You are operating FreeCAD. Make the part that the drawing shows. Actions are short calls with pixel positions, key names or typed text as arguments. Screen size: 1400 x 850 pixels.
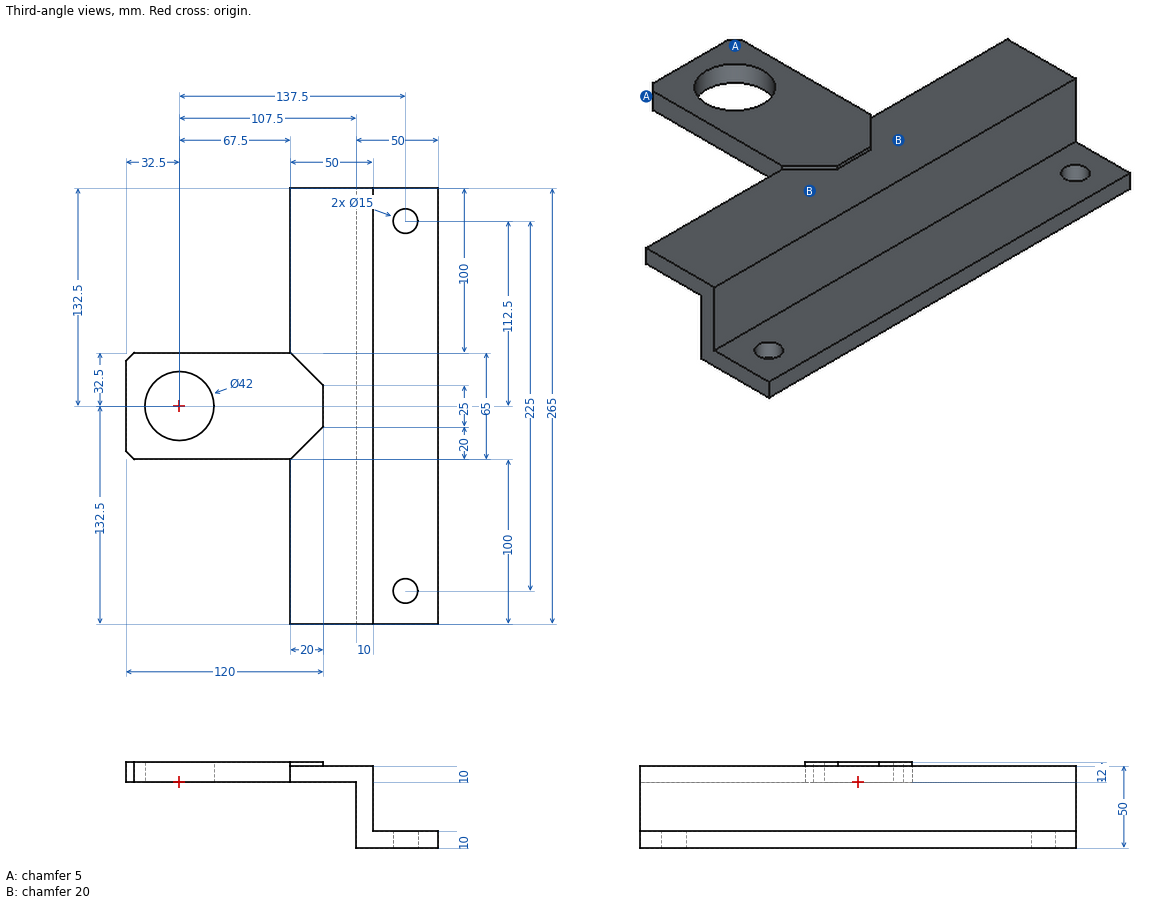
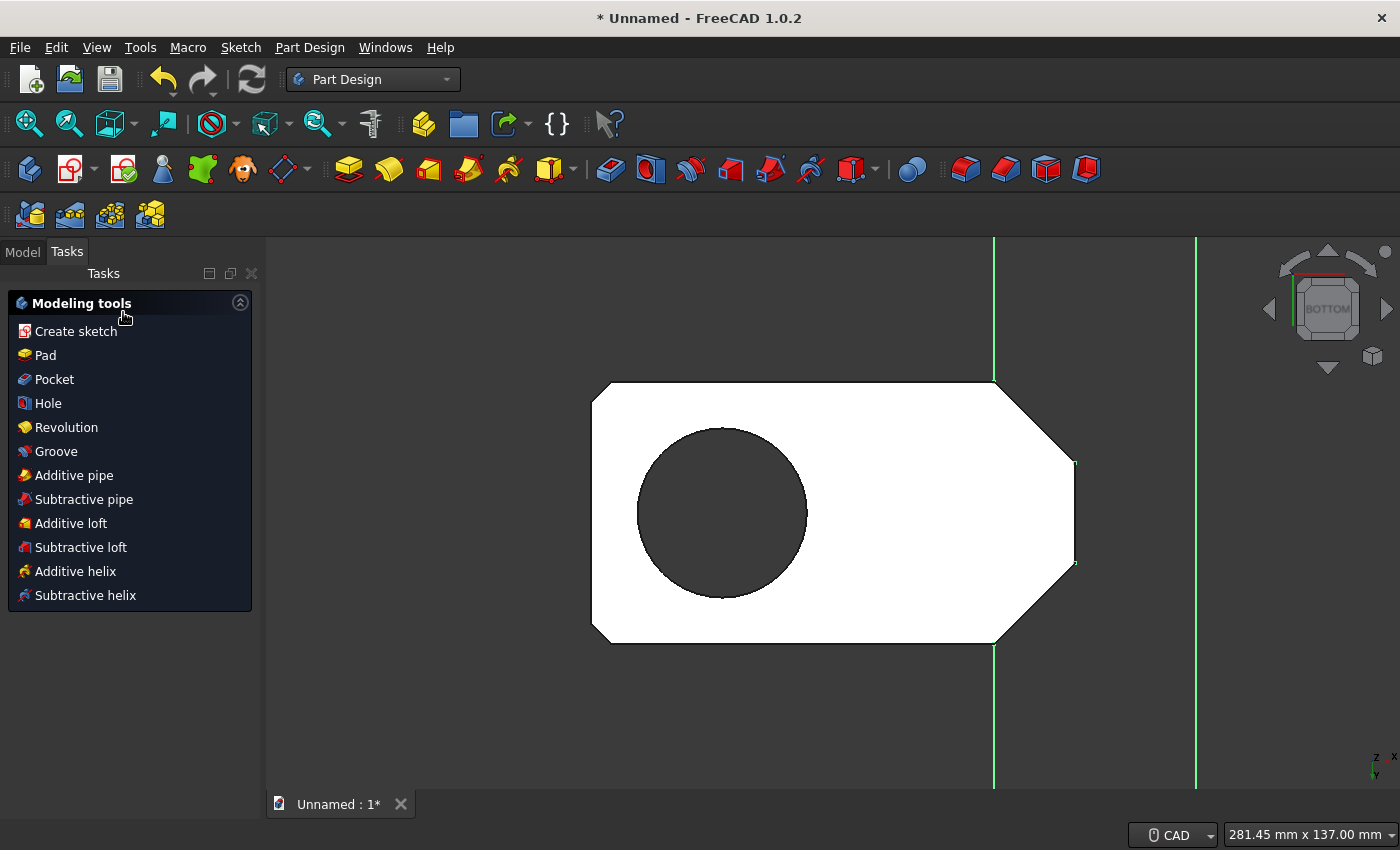
click(350, 170)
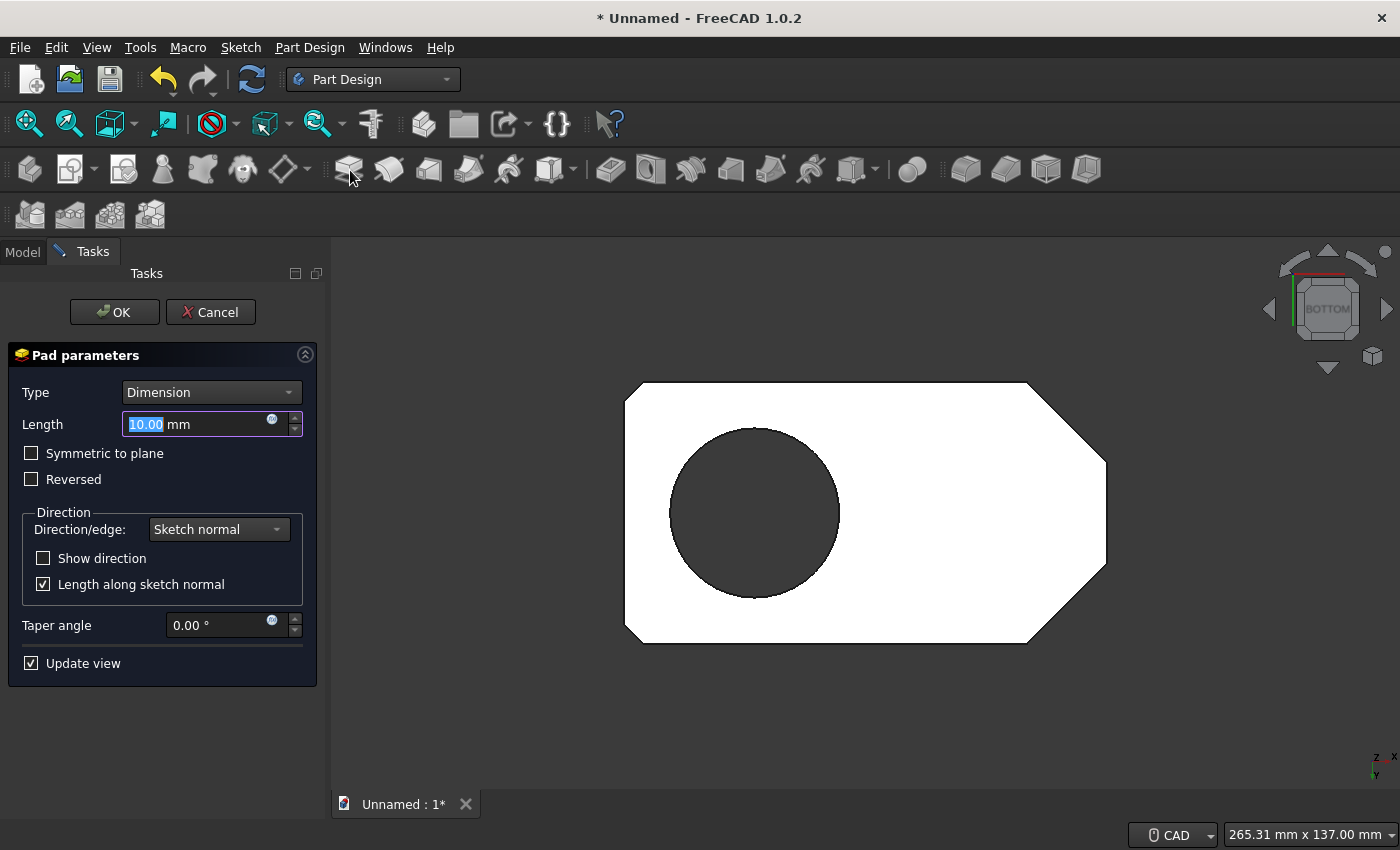
text(10)
key(Tab)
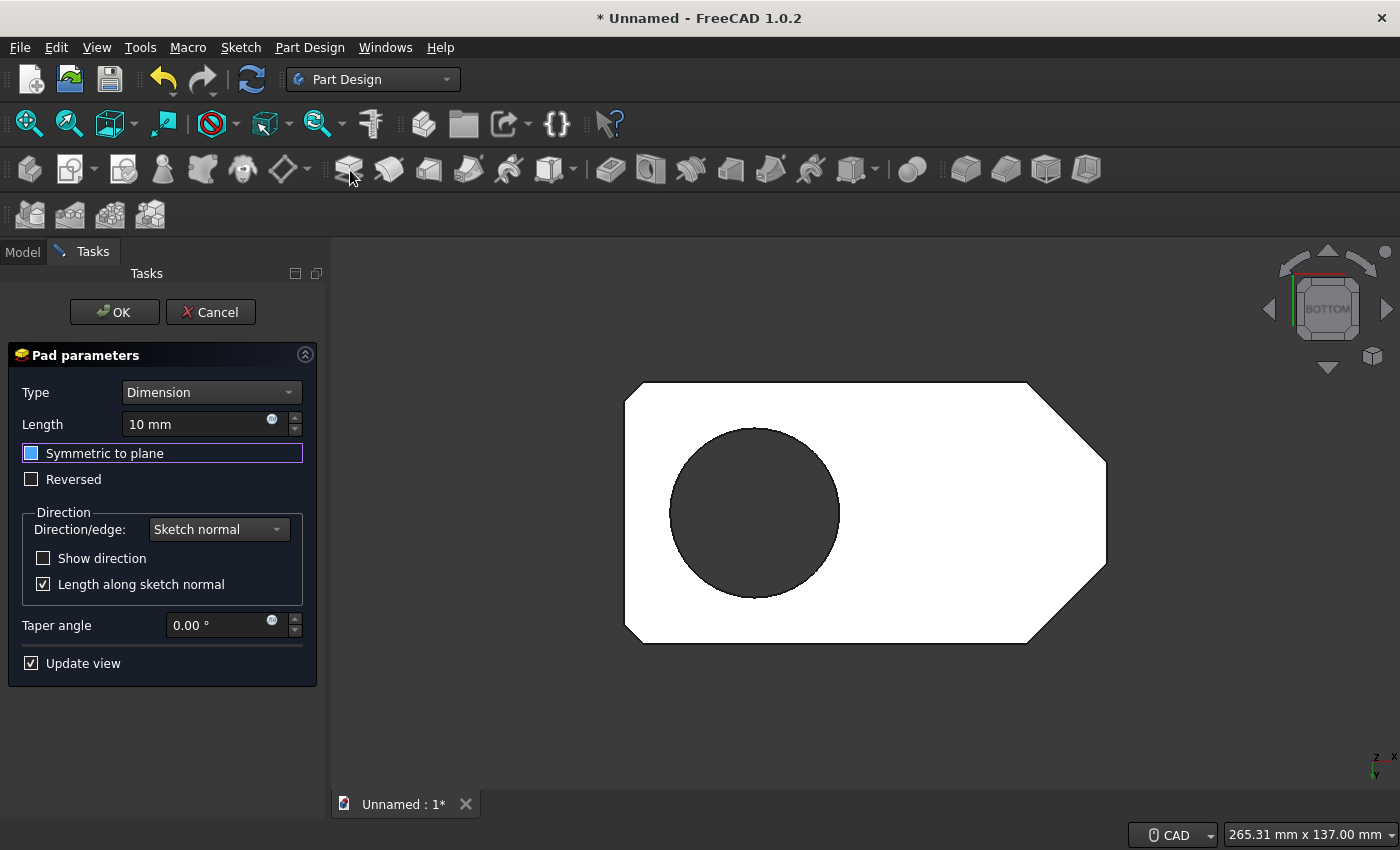
click(30, 479)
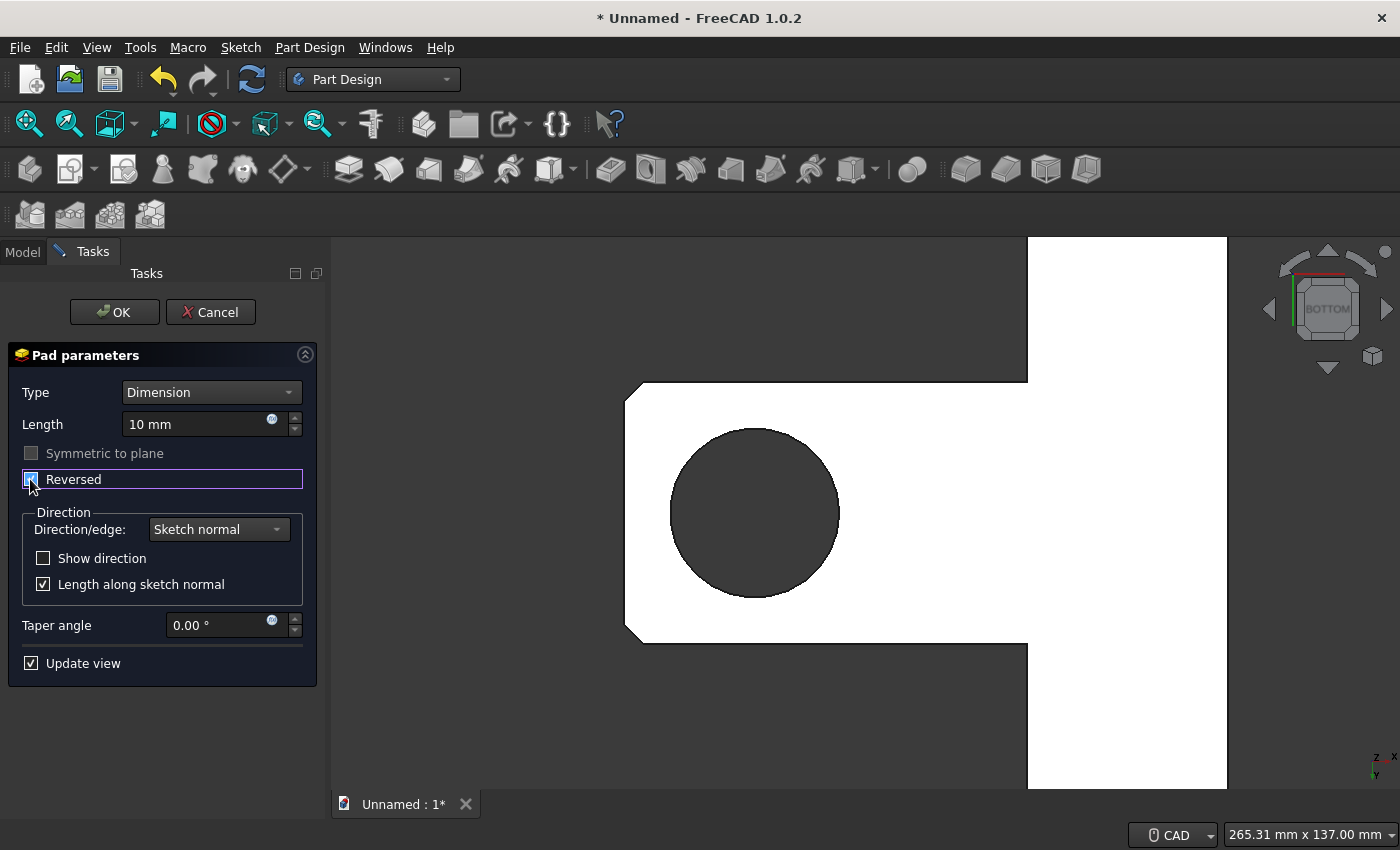
click(115, 312)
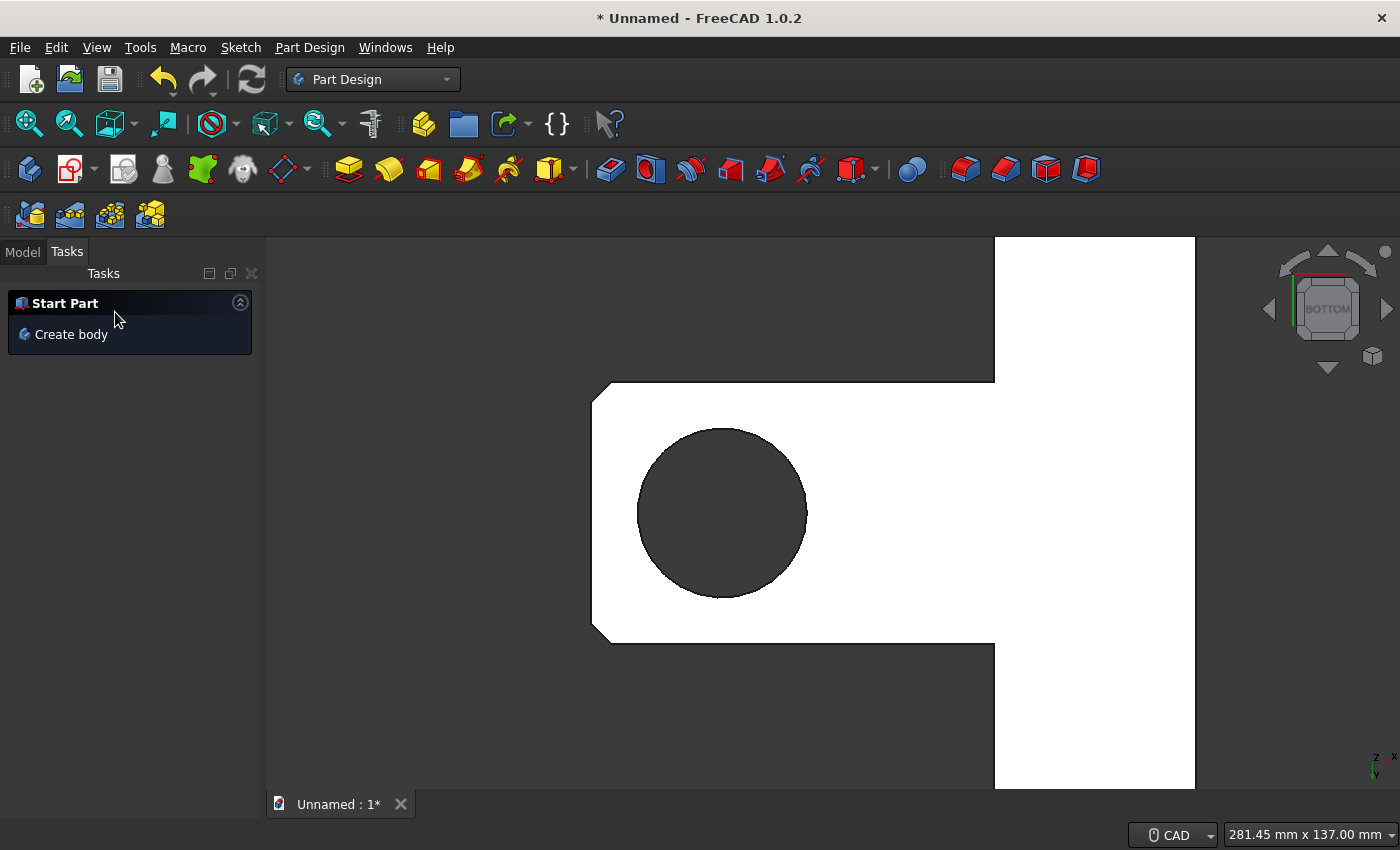
key(v)
key(f)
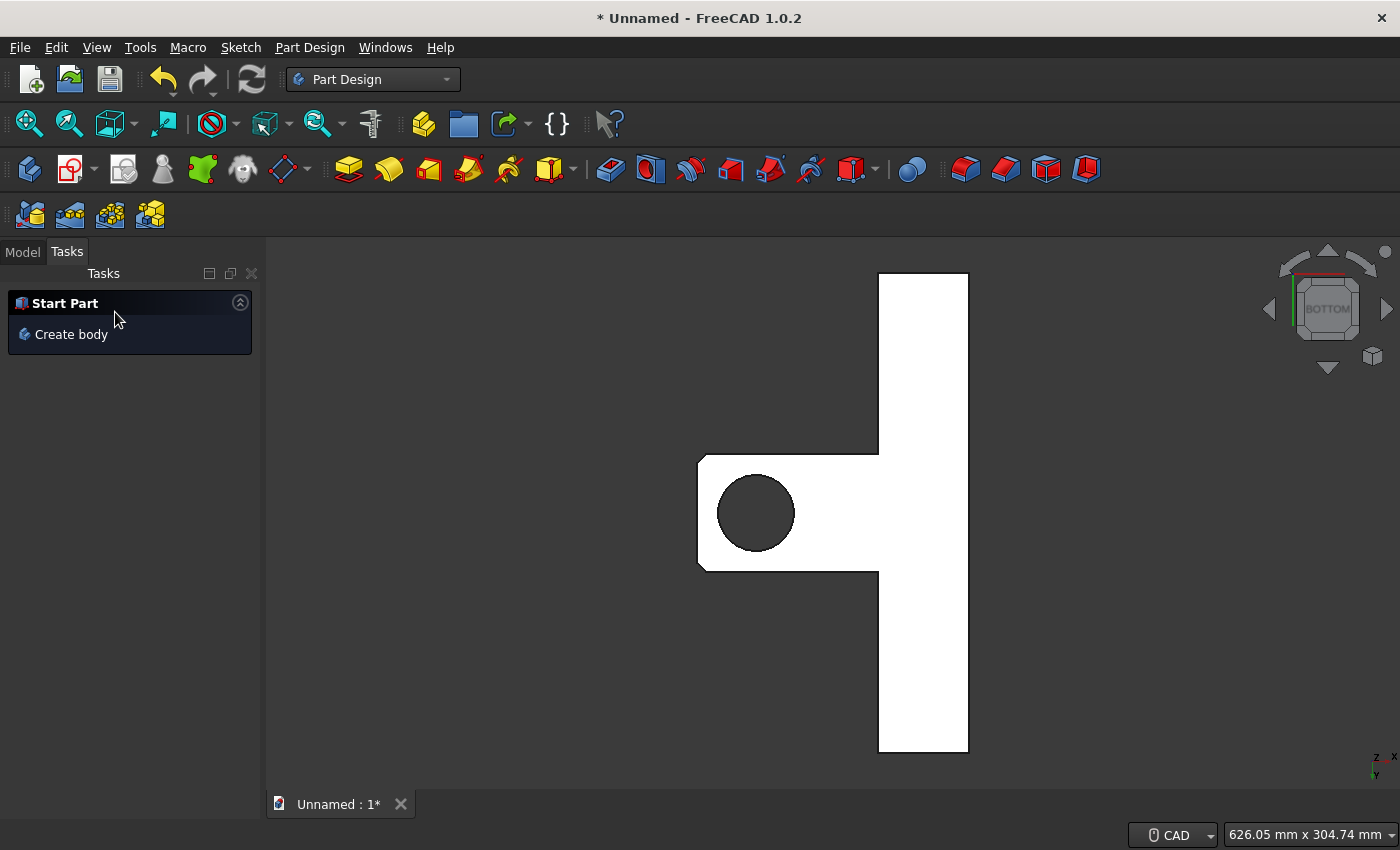
key(0)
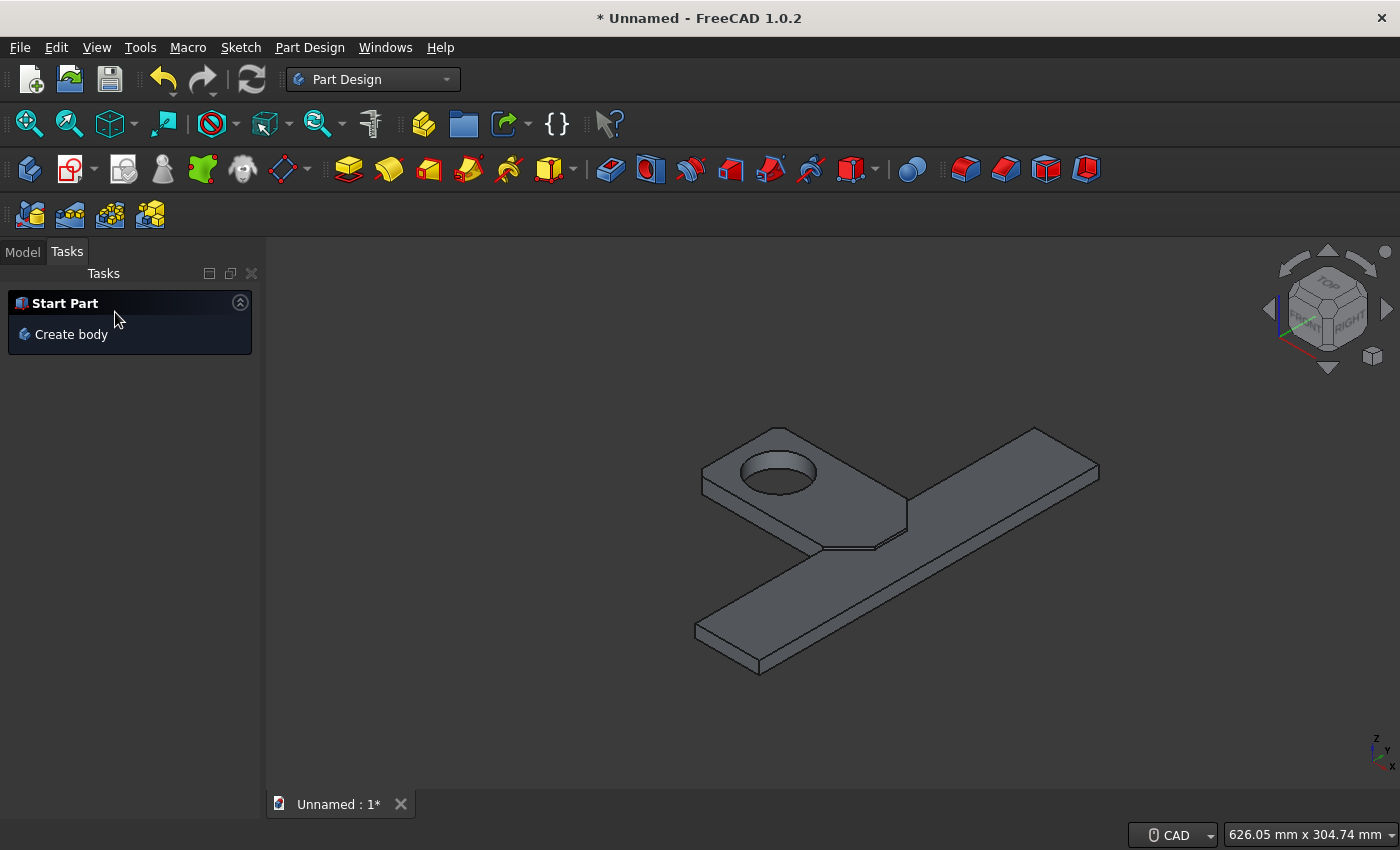
click(994, 487)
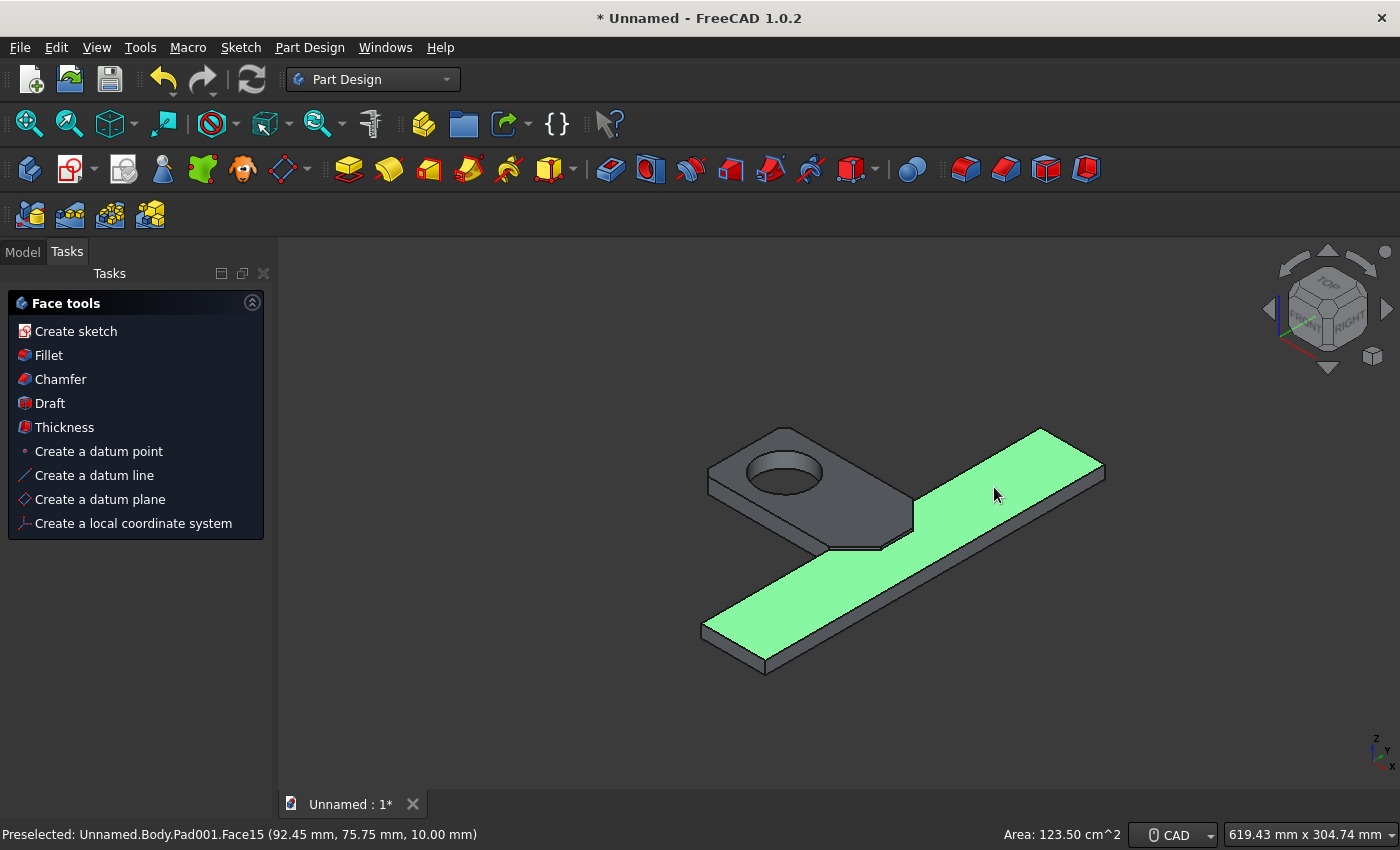
click(70, 170)